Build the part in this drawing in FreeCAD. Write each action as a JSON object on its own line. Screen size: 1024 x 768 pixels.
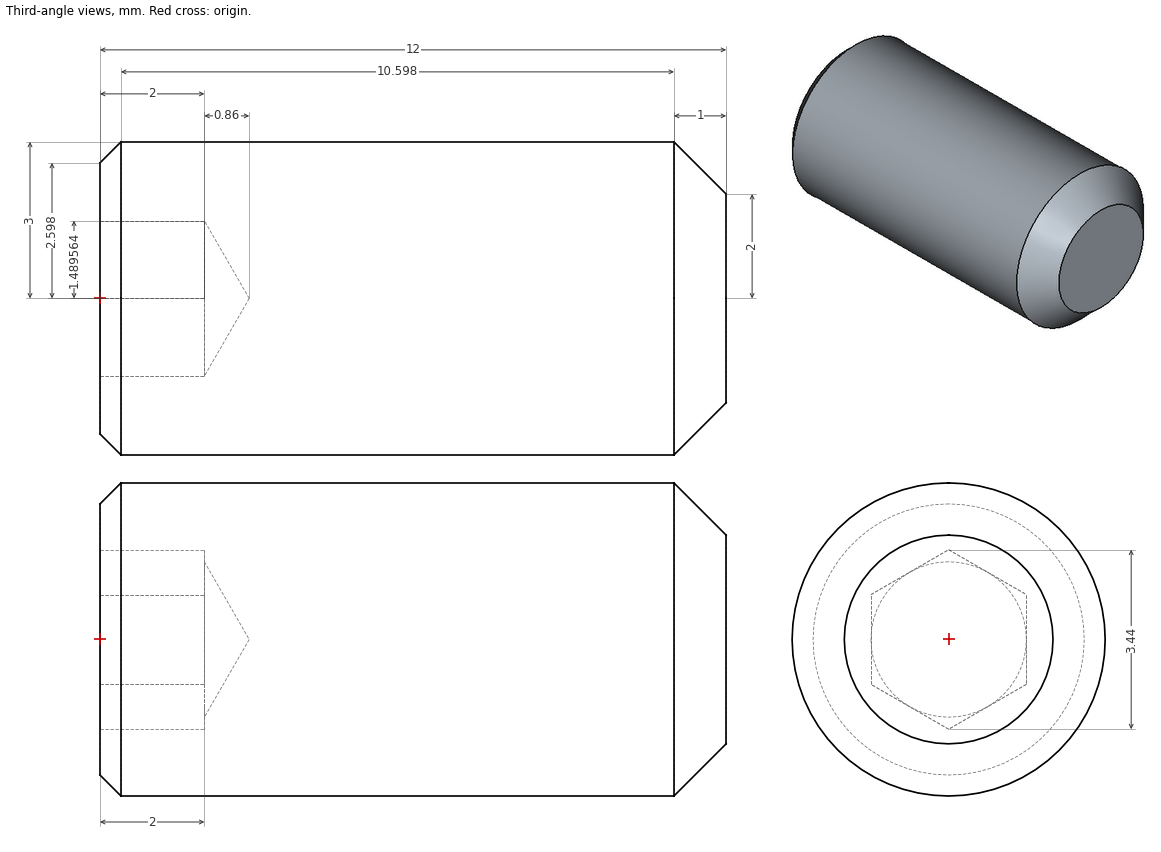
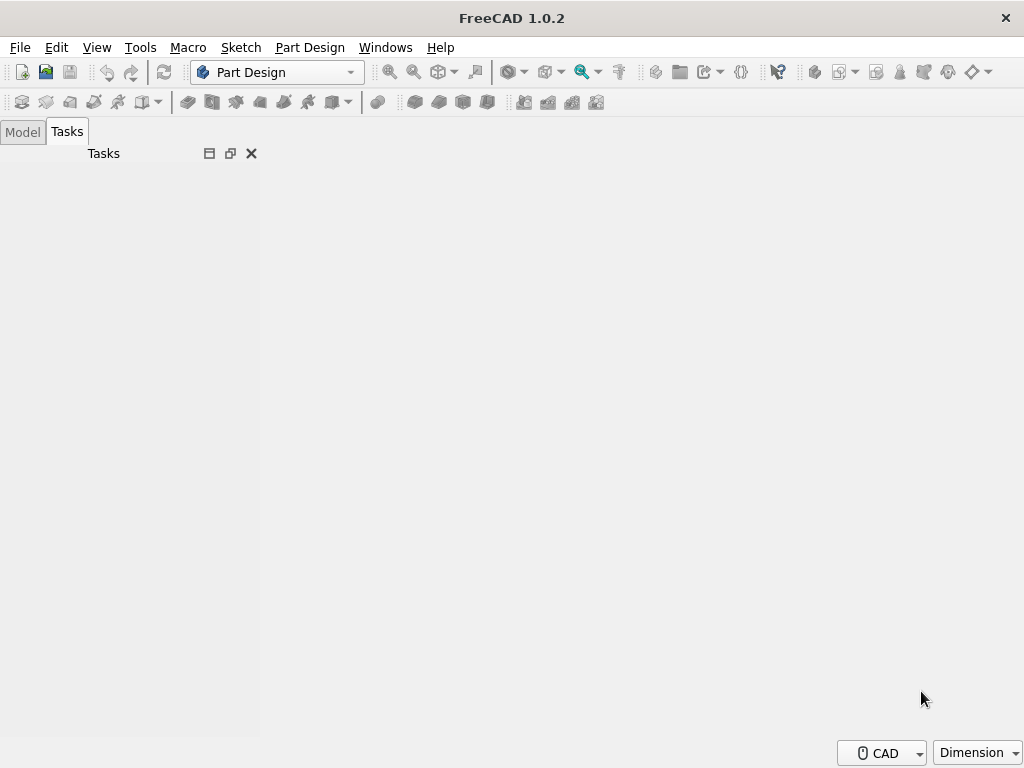
{"action": "key", "text": "ctrl+n"}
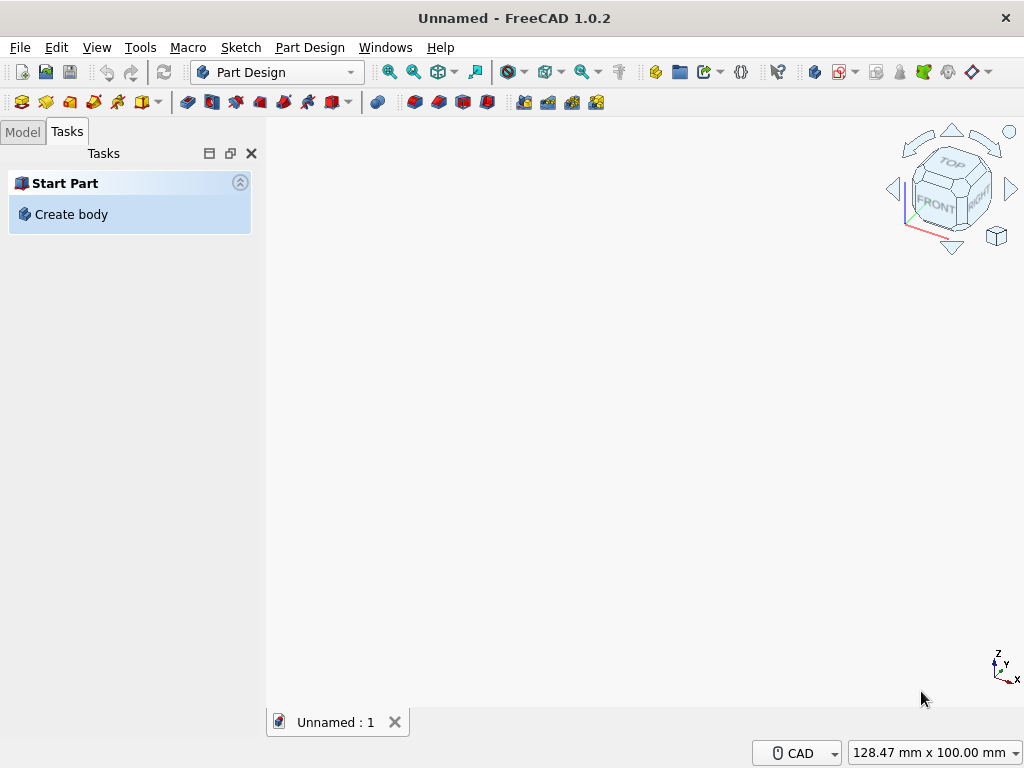
{"action": "left_click", "coordinate": [840, 72]}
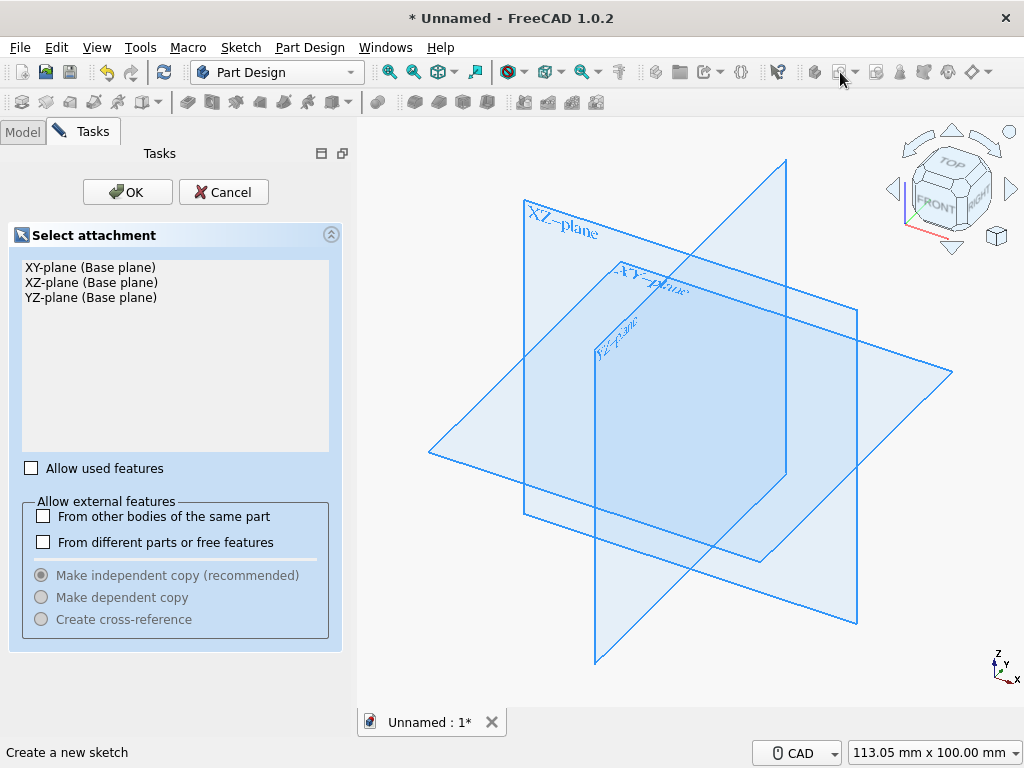
{"action": "left_click", "coordinate": [82, 268]}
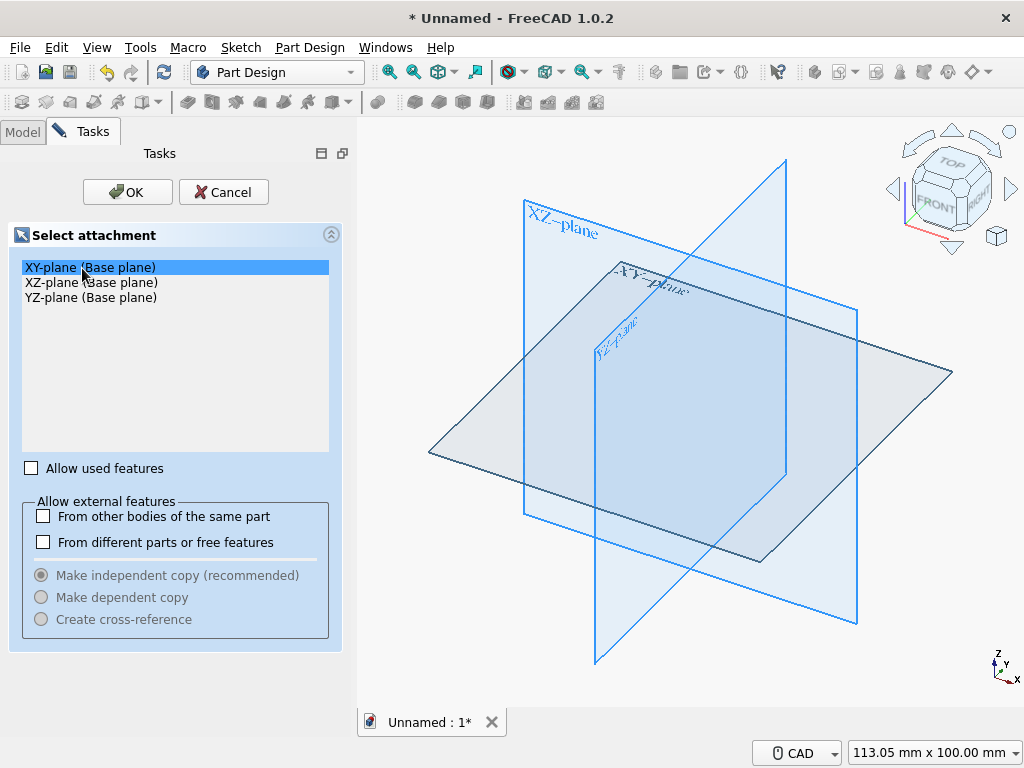
{"action": "left_click", "coordinate": [128, 192]}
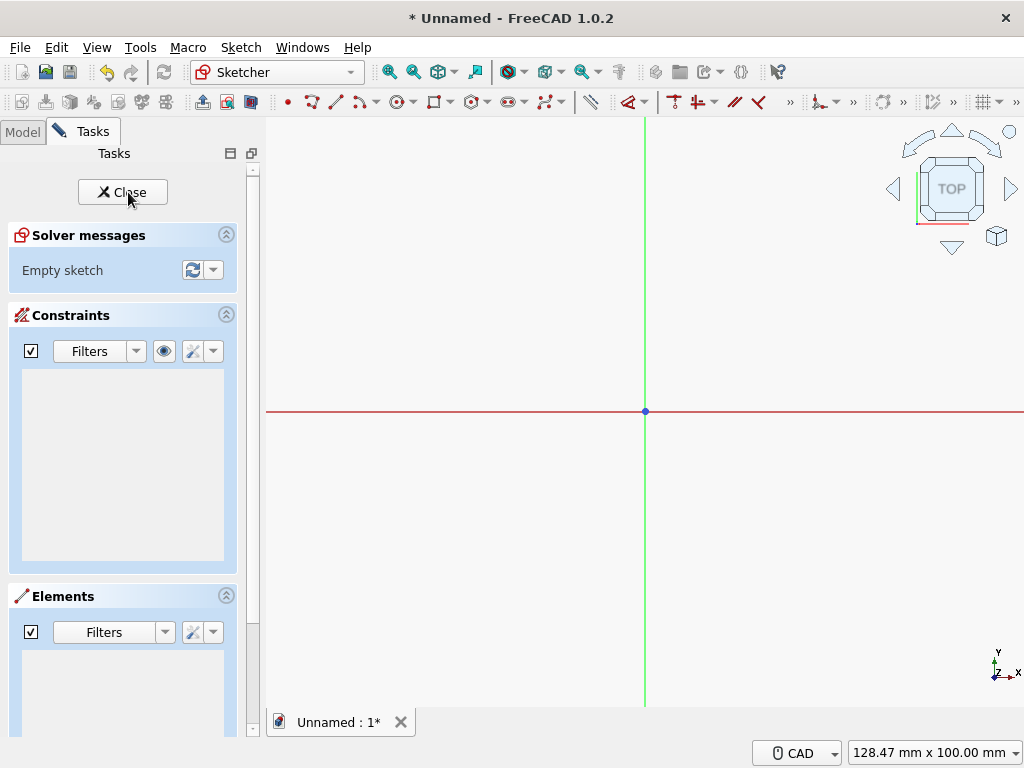
{"action": "scroll", "coordinate": [701, 401], "scroll_direction": "up", "scroll_amount": 9}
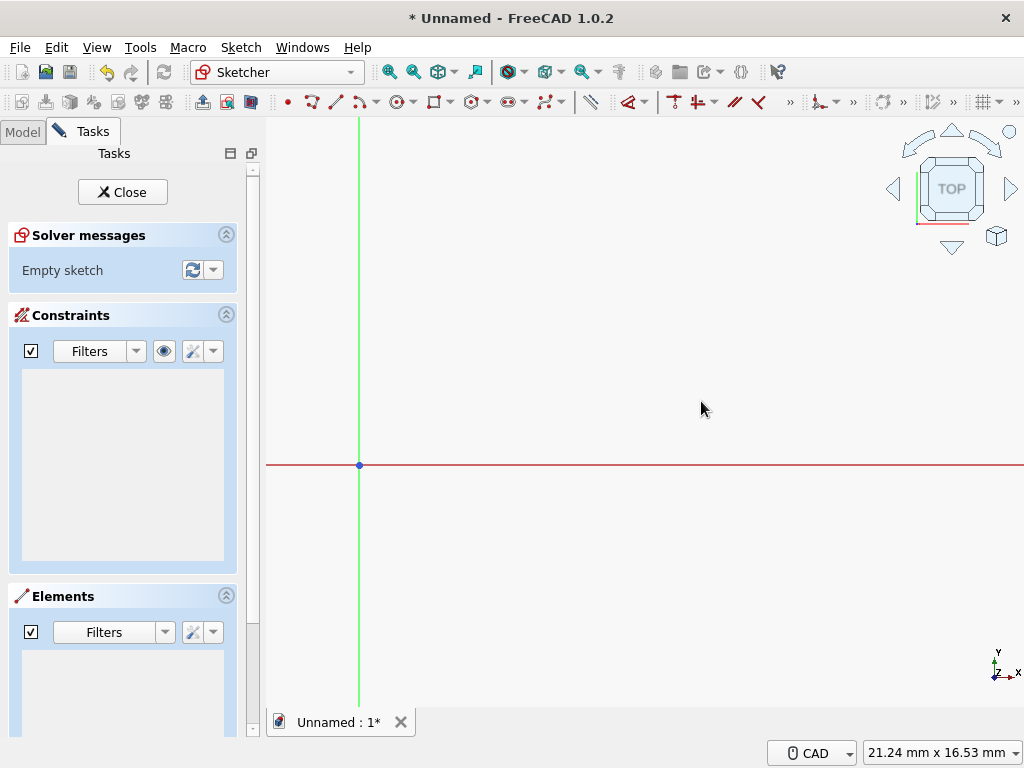
{"action": "key", "text": "g m"}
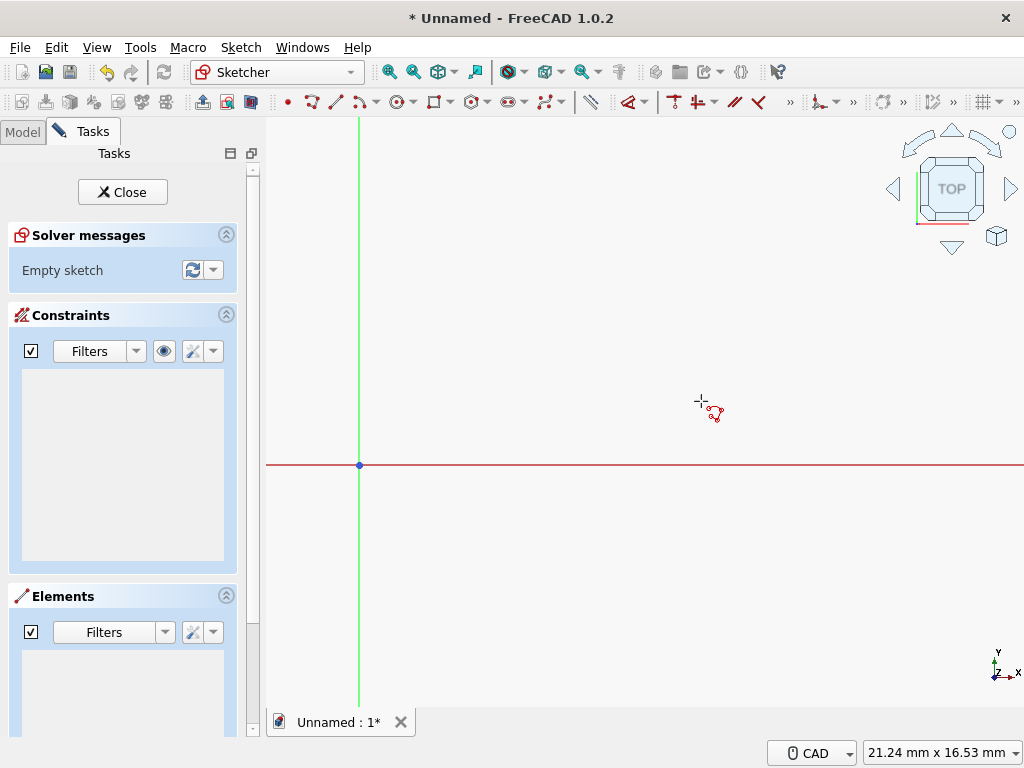
{"action": "left_click", "coordinate": [359, 465]}
{"action": "left_click", "coordinate": [788, 456]}
{"action": "left_click", "coordinate": [788, 394]}
{"action": "left_click", "coordinate": [752, 358]}
{"action": "left_click", "coordinate": [374, 358]}
{"action": "left_click", "coordinate": [368, 372]}
{"action": "left_click", "coordinate": [359, 465]}
{"action": "key", "text": "Escape"}
{"action": "key", "text": "Escape"}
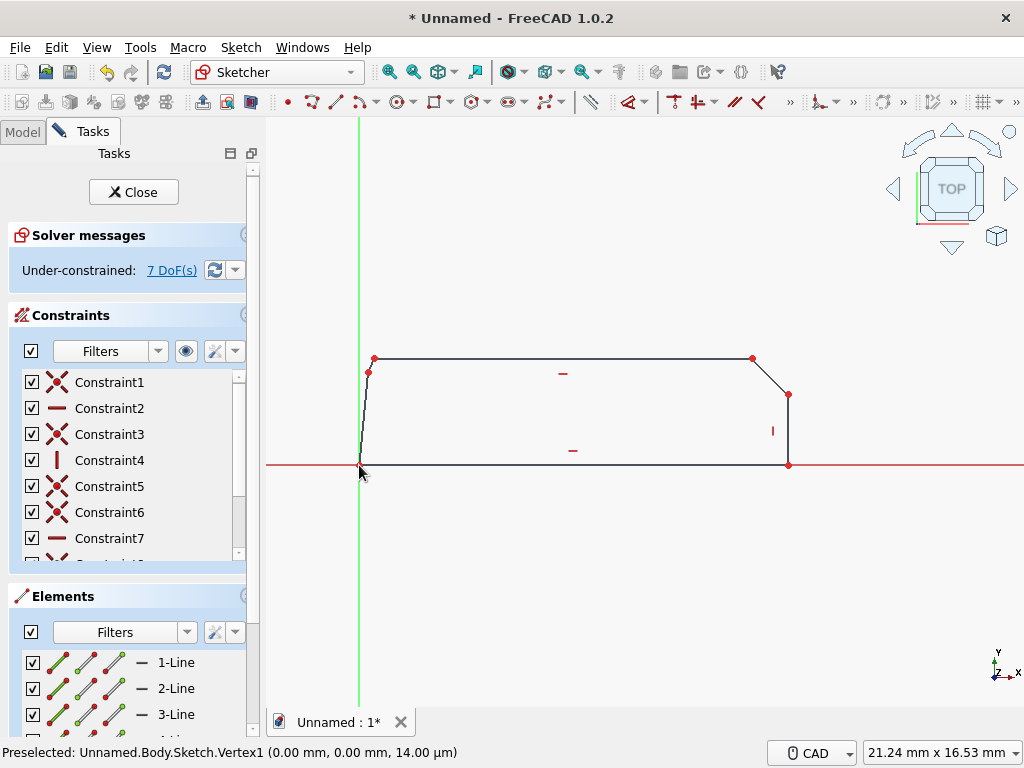
{"action": "left_click", "coordinate": [362, 437]}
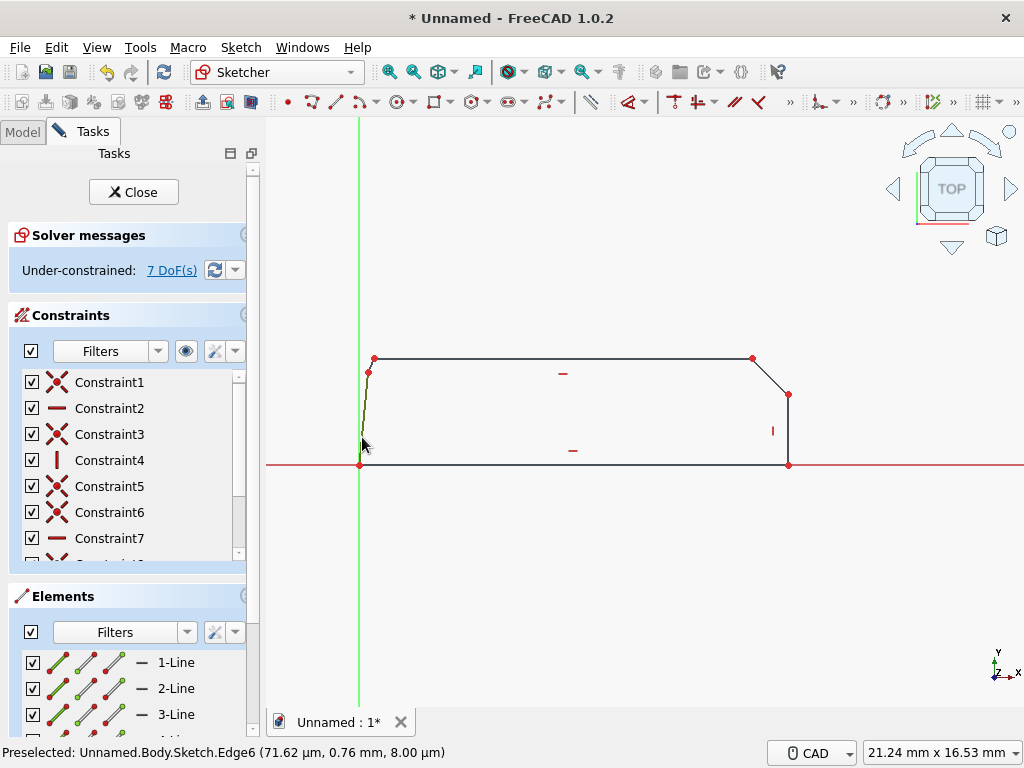
{"action": "key", "text": "v"}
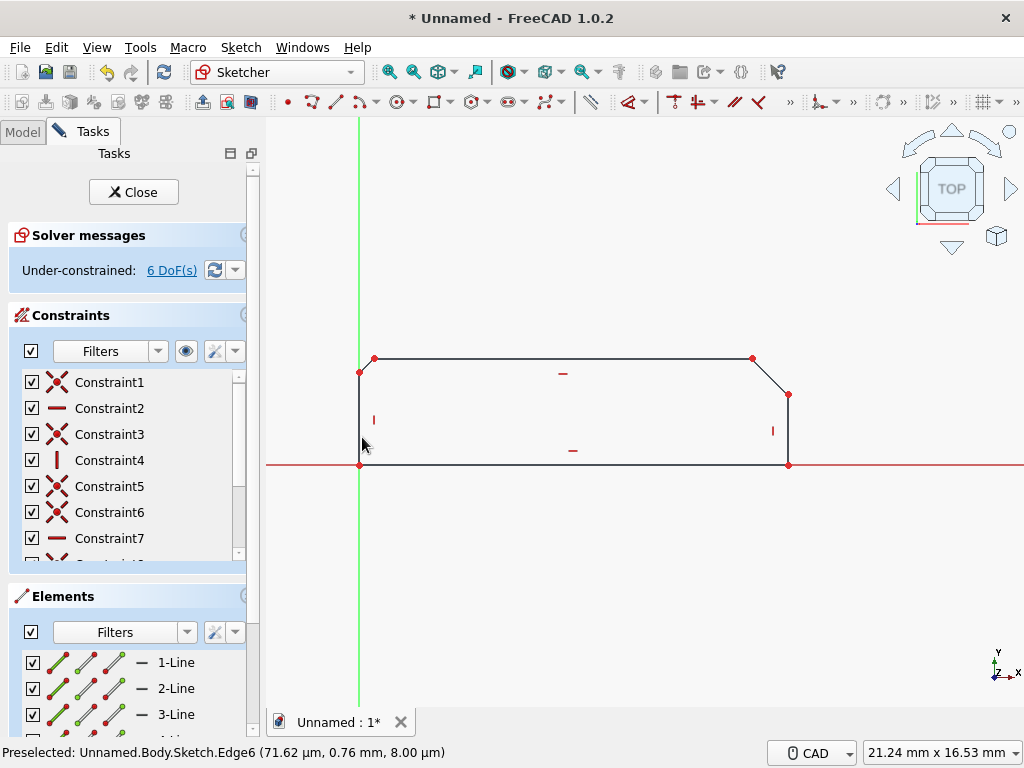
{"action": "key", "text": "d"}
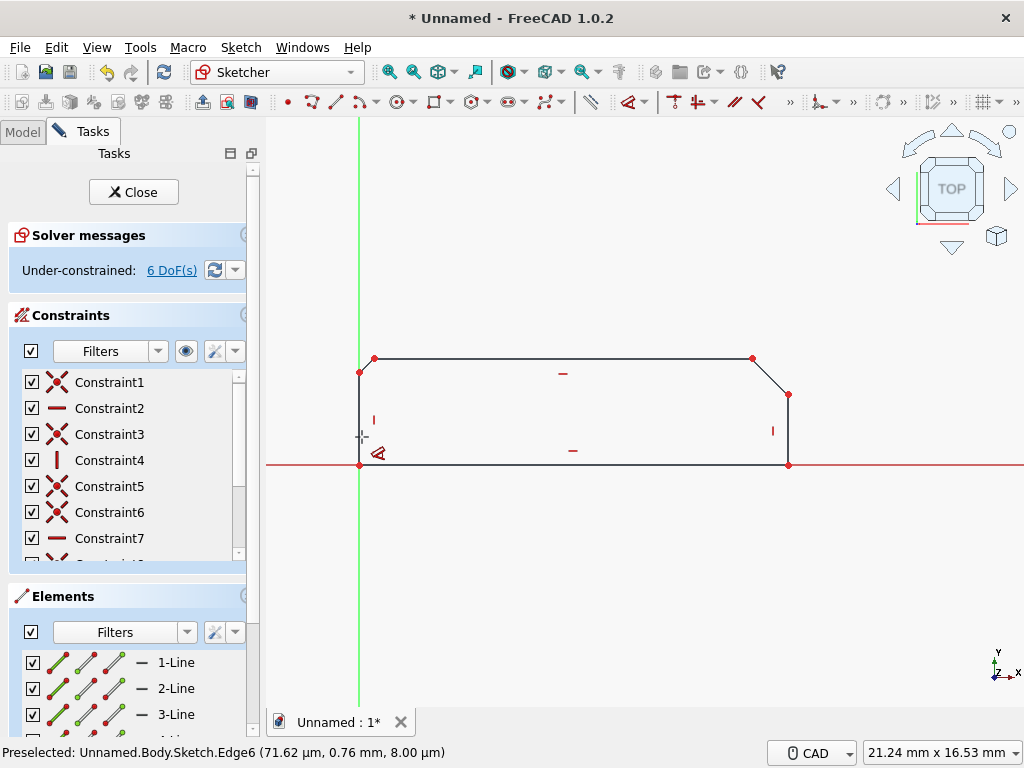
{"action": "left_click", "coordinate": [788, 444]}
{"action": "left_click", "coordinate": [822, 430]}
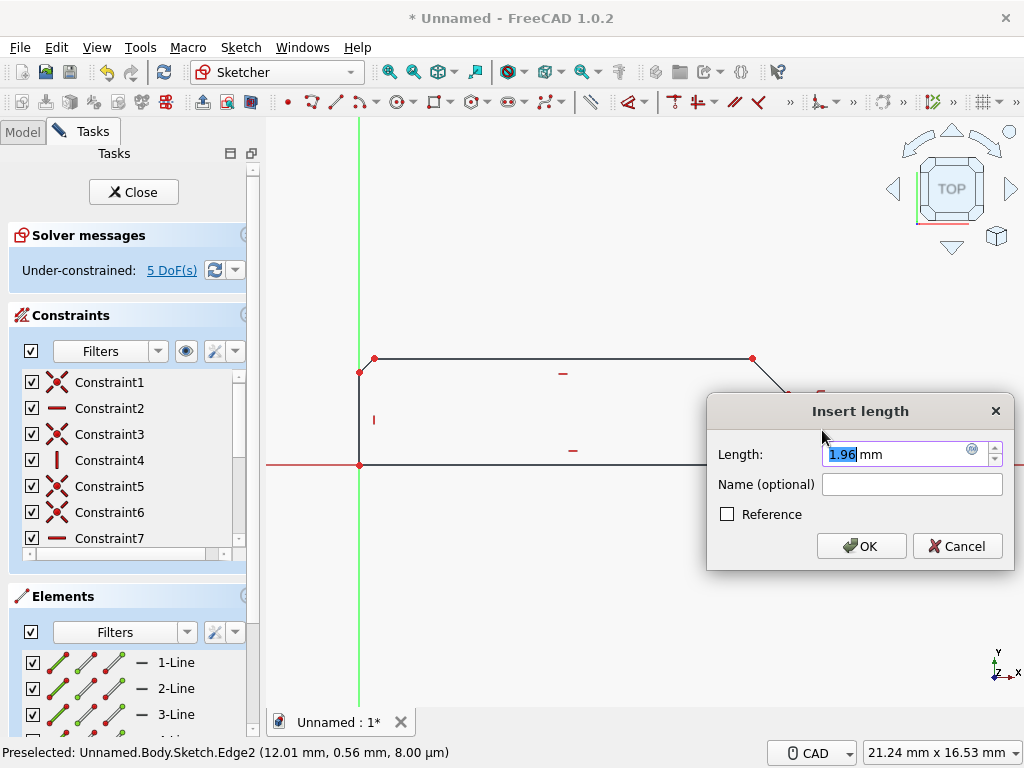
{"action": "type", "text": "2"}
{"action": "key", "text": "Return"}